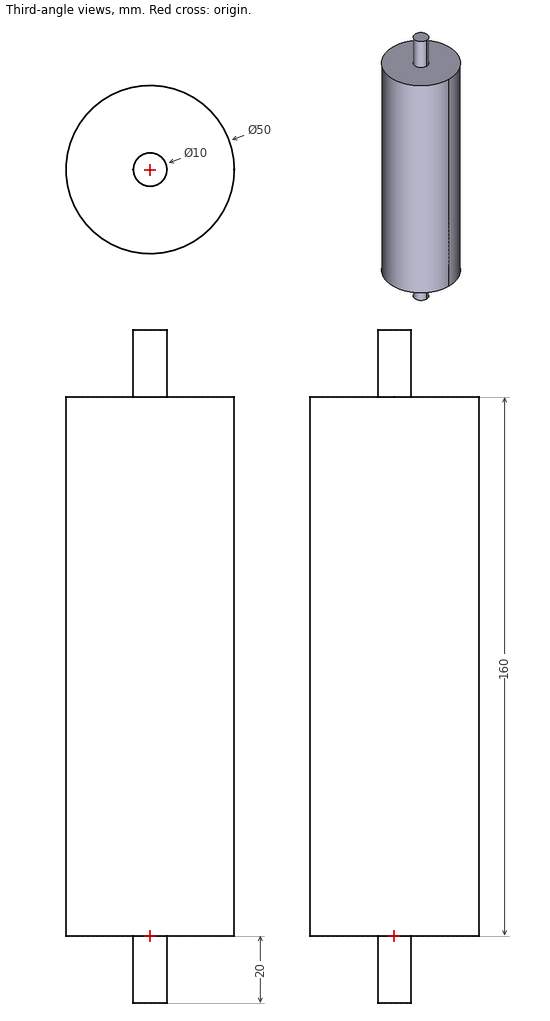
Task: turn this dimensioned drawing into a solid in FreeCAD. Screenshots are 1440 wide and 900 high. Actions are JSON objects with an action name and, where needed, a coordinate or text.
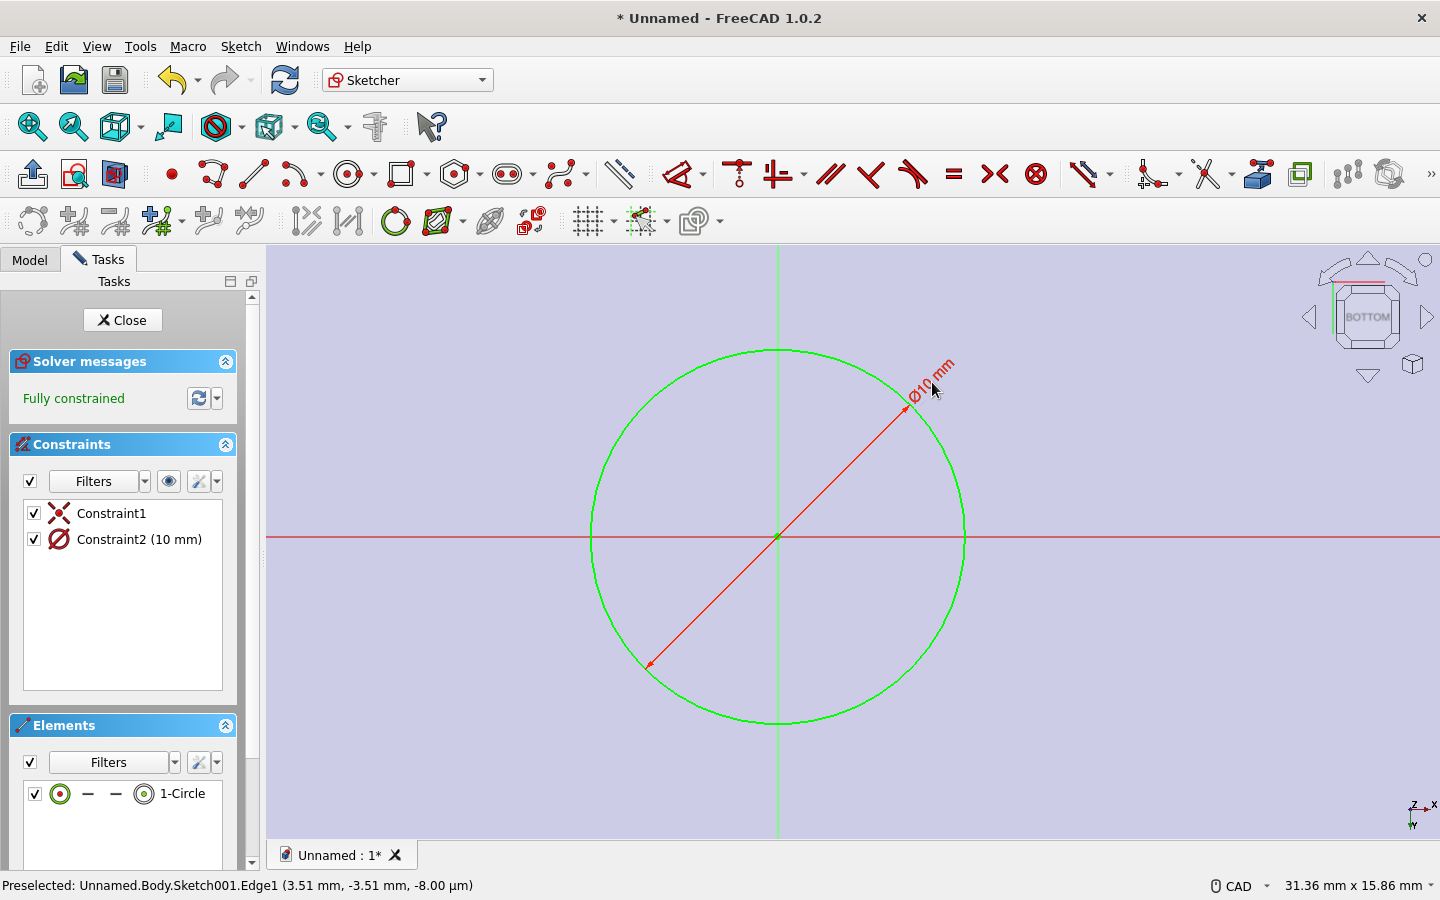
{"action": "left_click", "coordinate": [123, 320]}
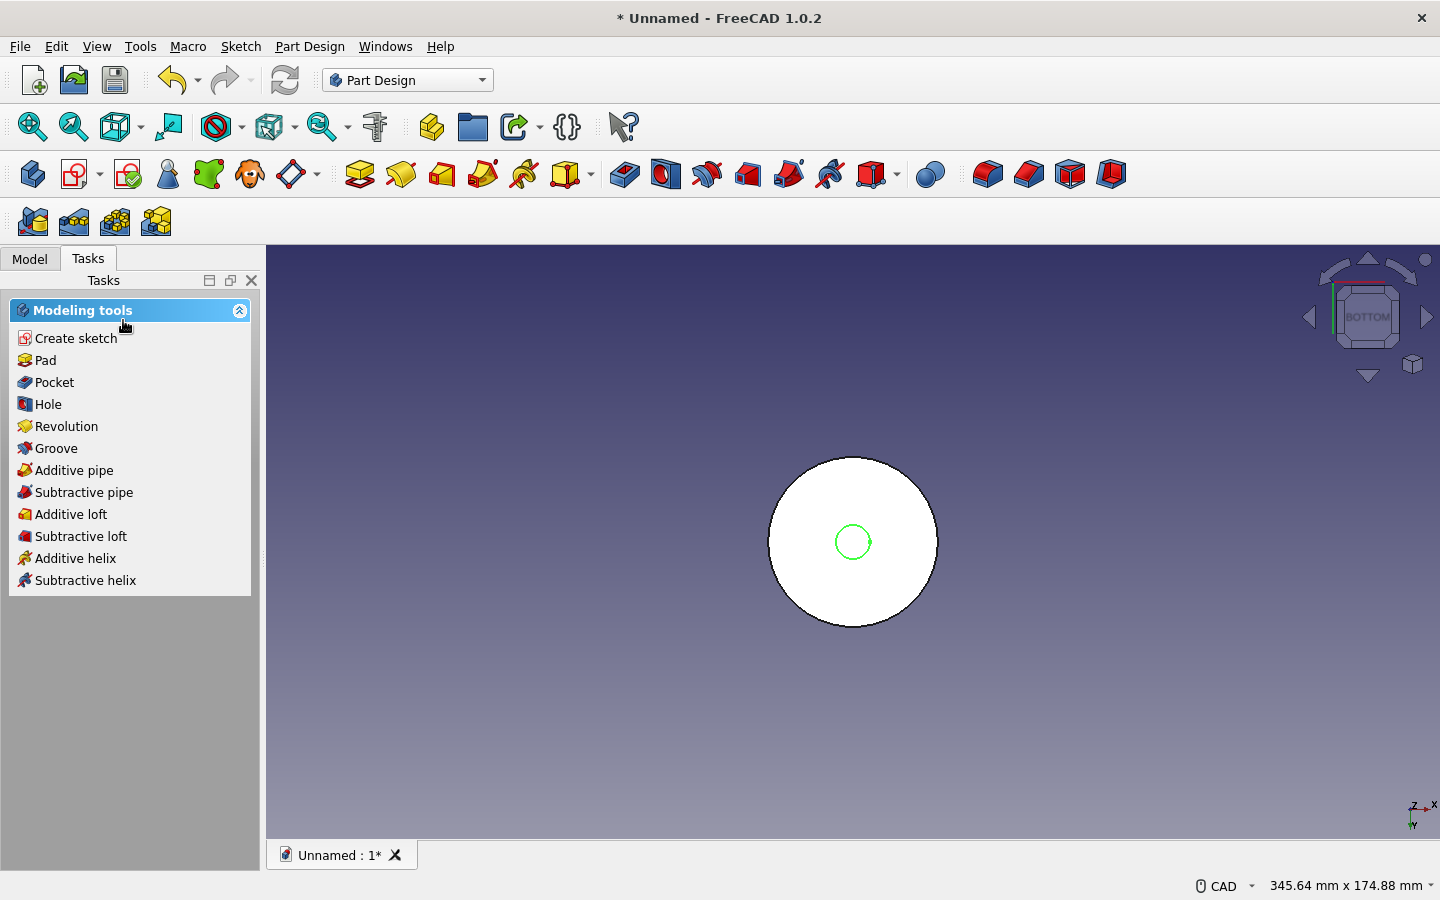
{"action": "left_click", "coordinate": [360, 174]}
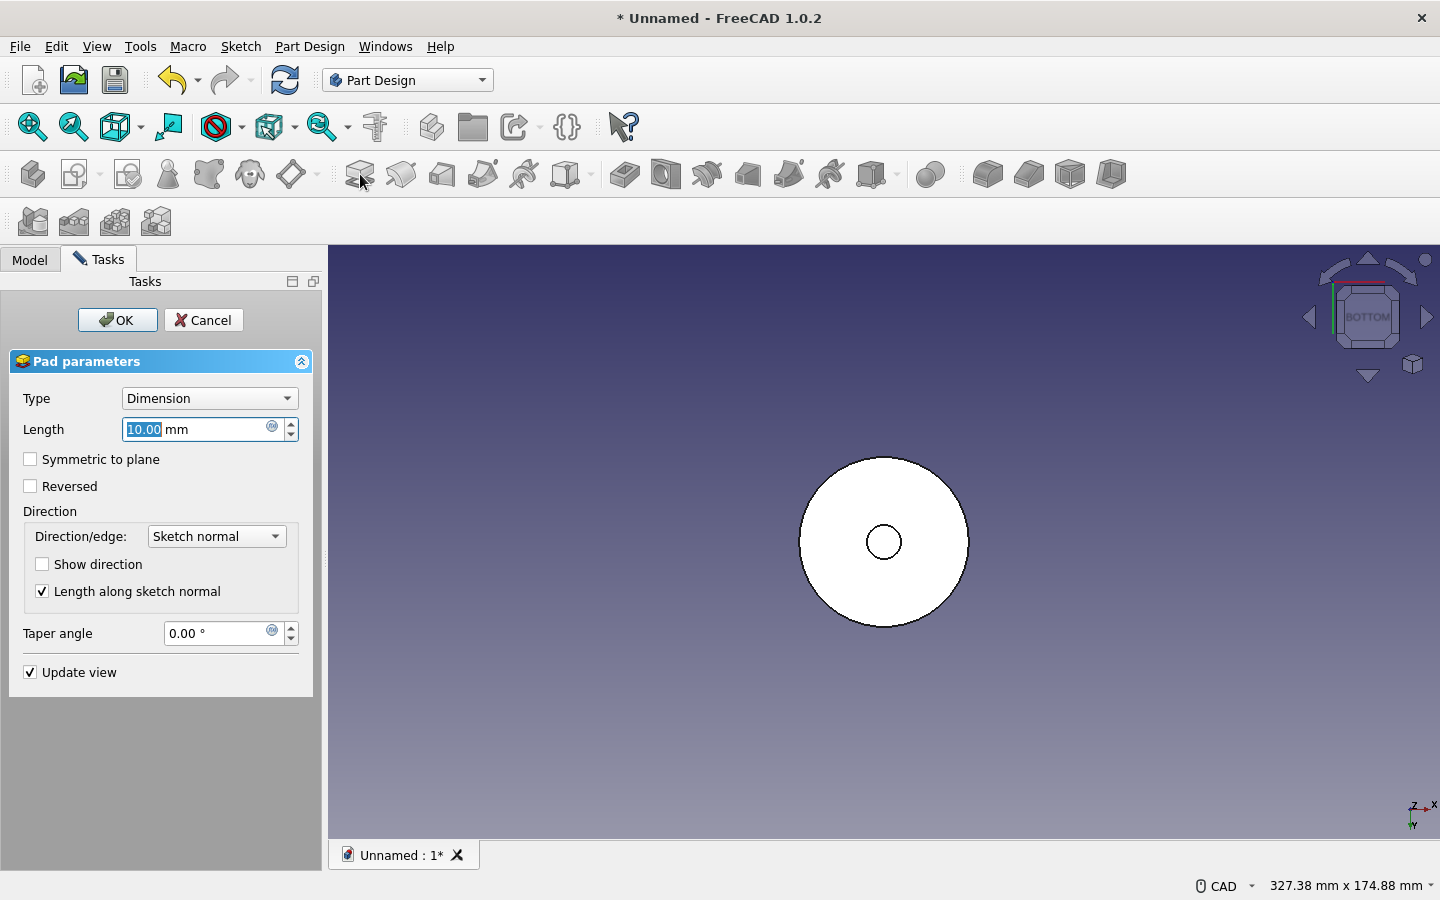
{"action": "type", "text": "20"}
{"action": "key", "text": "Tab"}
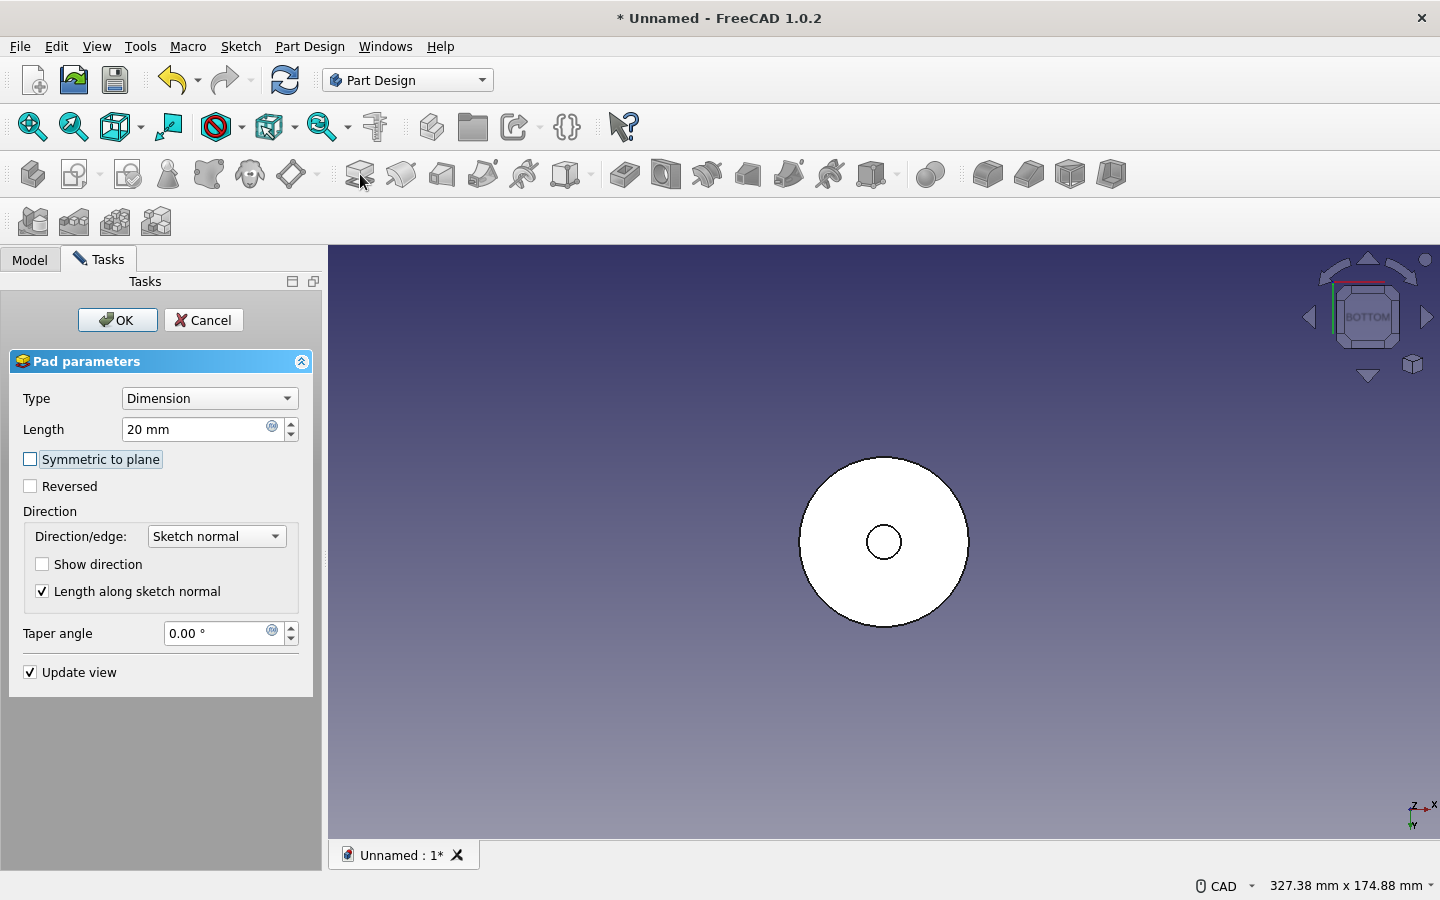
{"action": "left_click", "coordinate": [118, 320]}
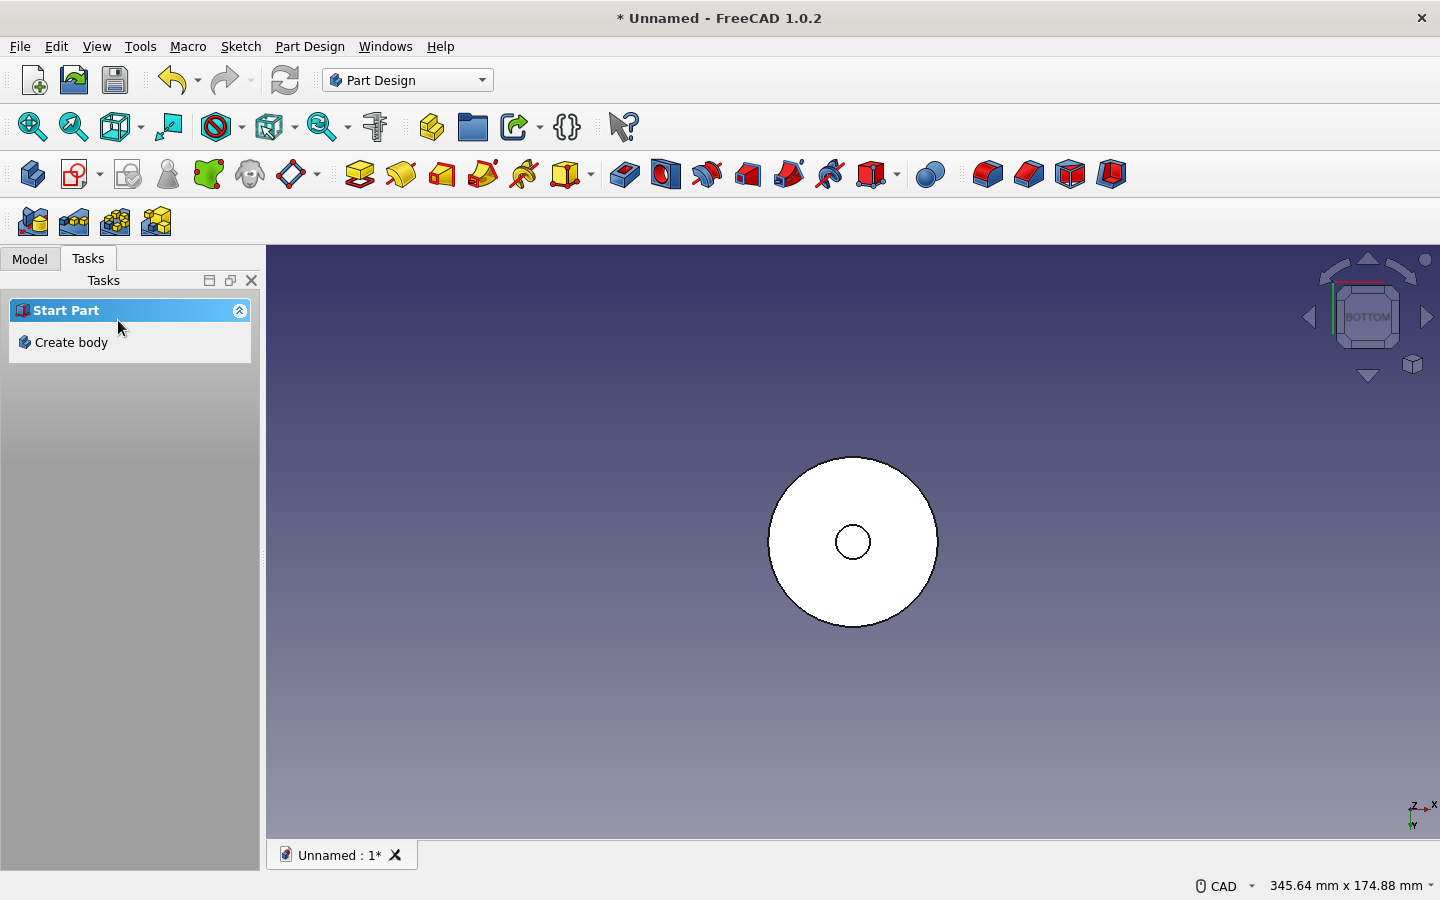
{"action": "key", "text": "v f"}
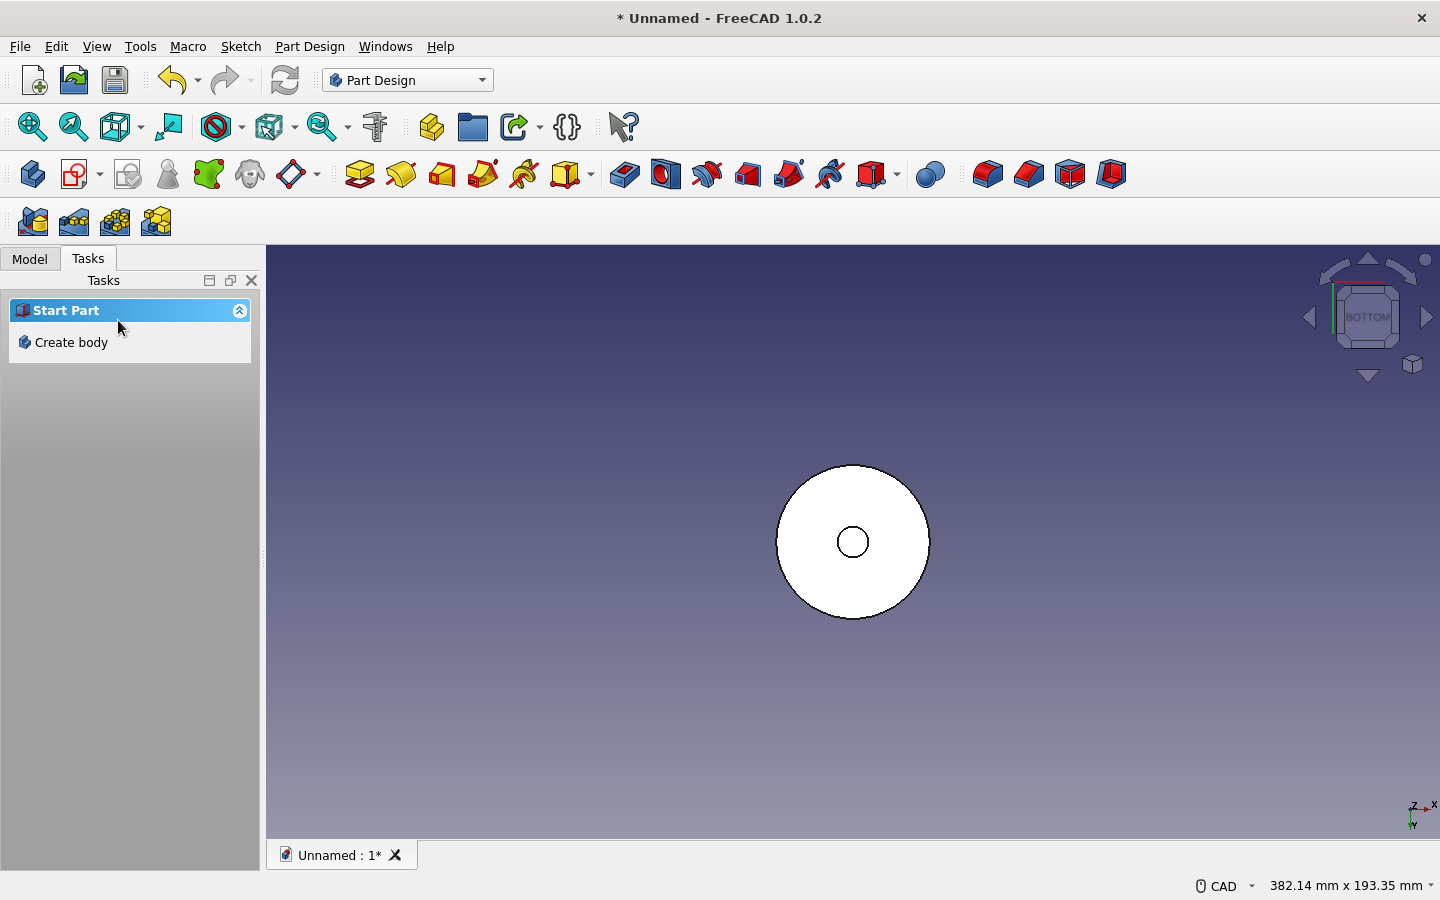
{"action": "left_click", "coordinate": [30, 258]}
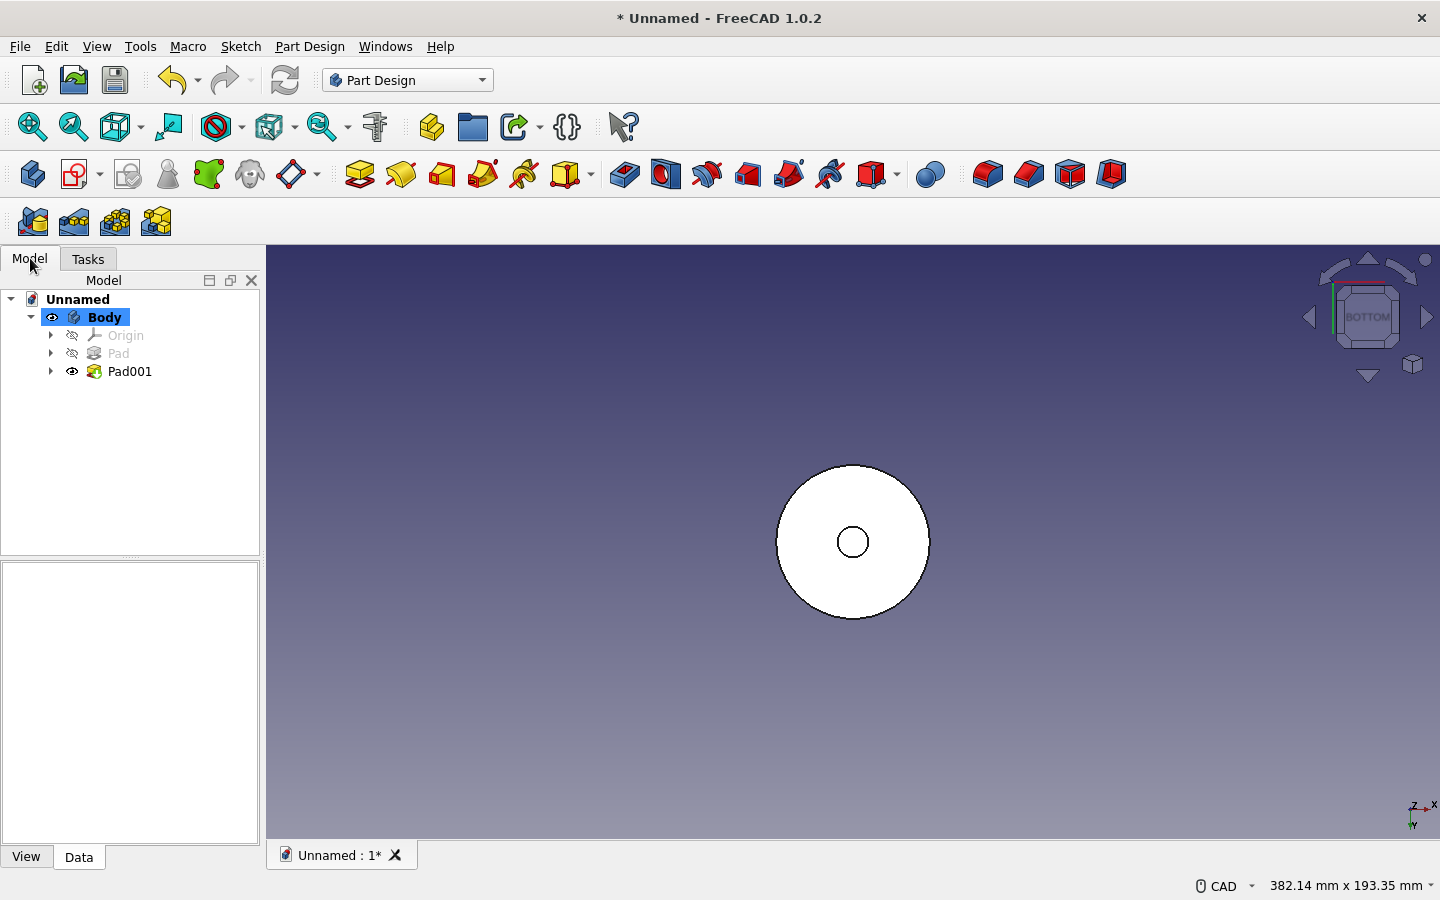
{"action": "left_click", "coordinate": [51, 335]}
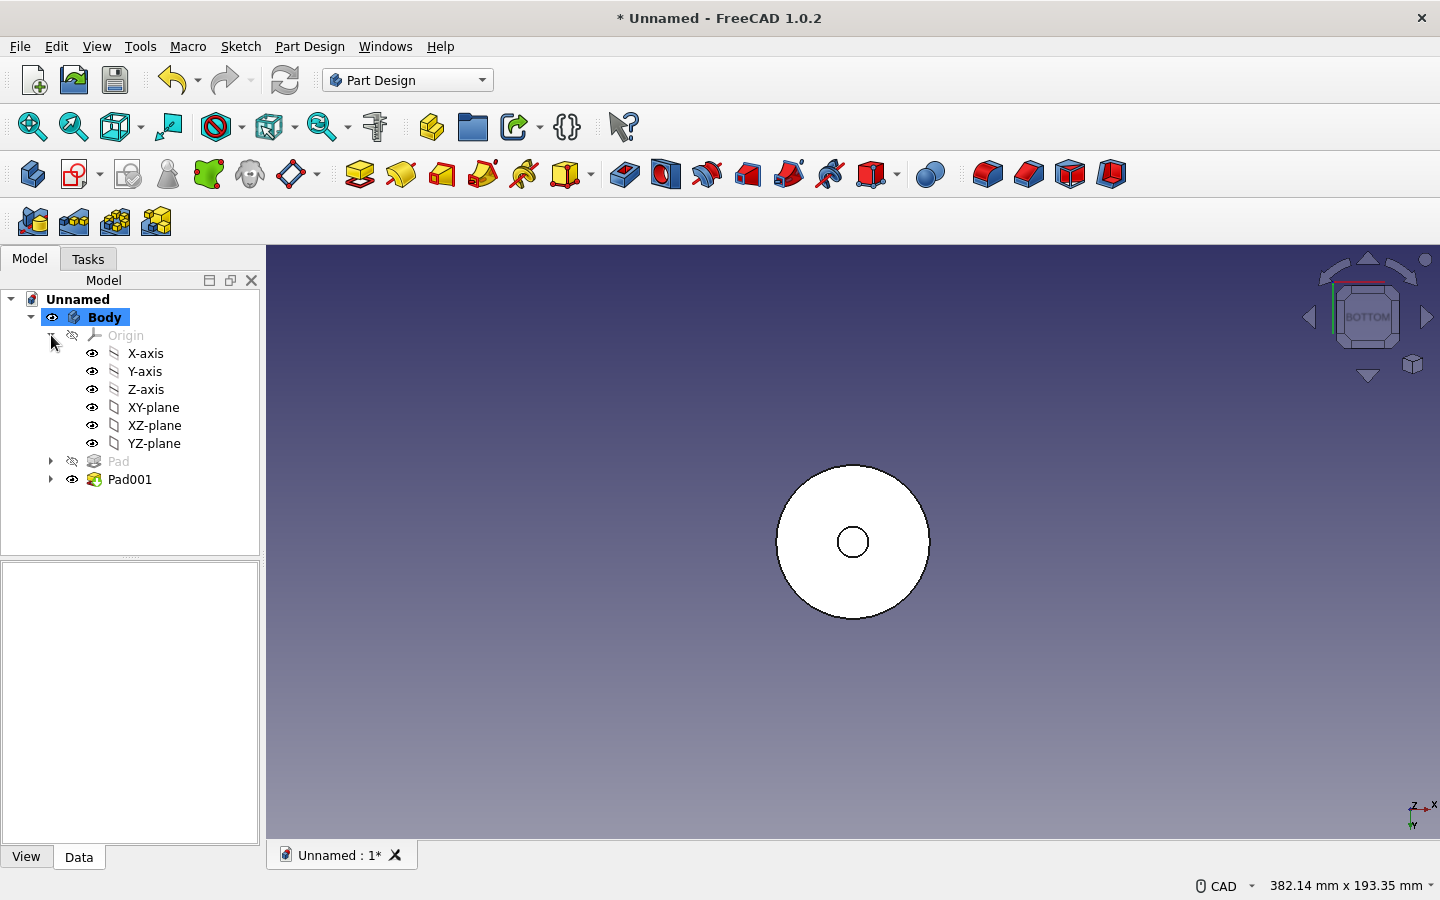
{"action": "left_click", "coordinate": [137, 407]}